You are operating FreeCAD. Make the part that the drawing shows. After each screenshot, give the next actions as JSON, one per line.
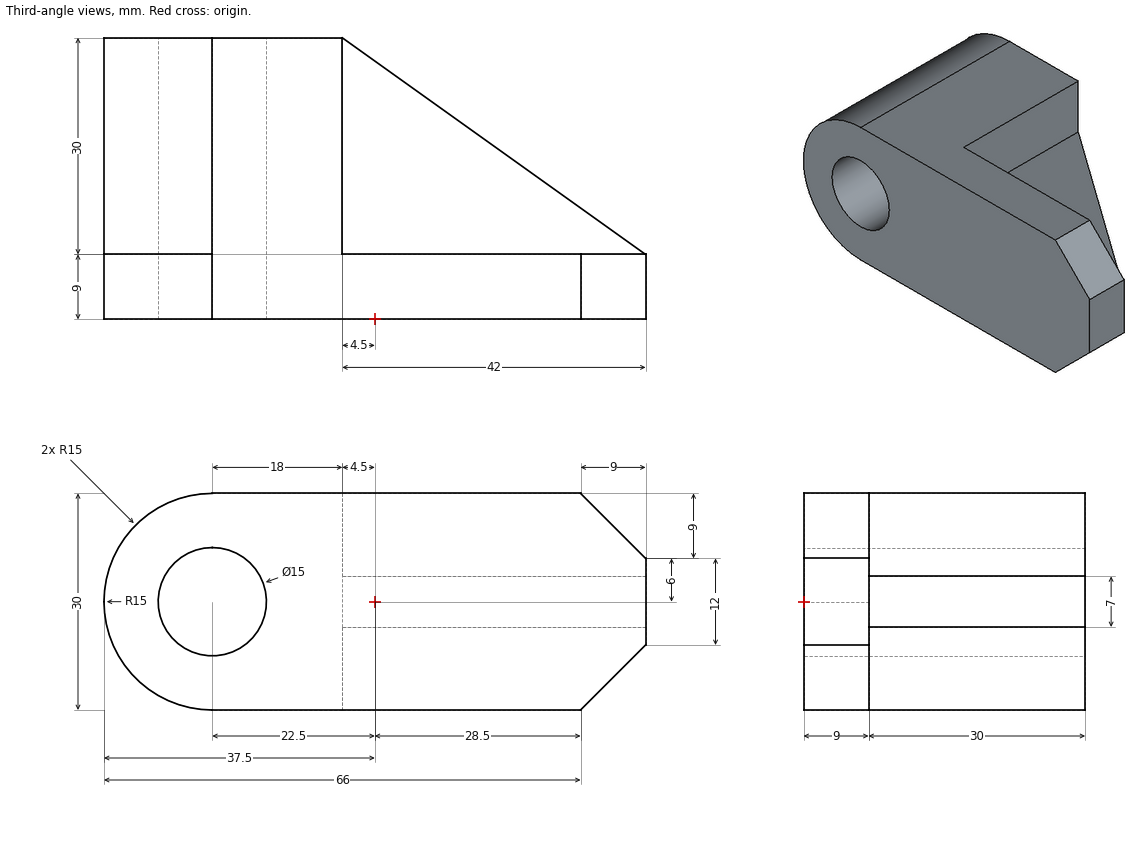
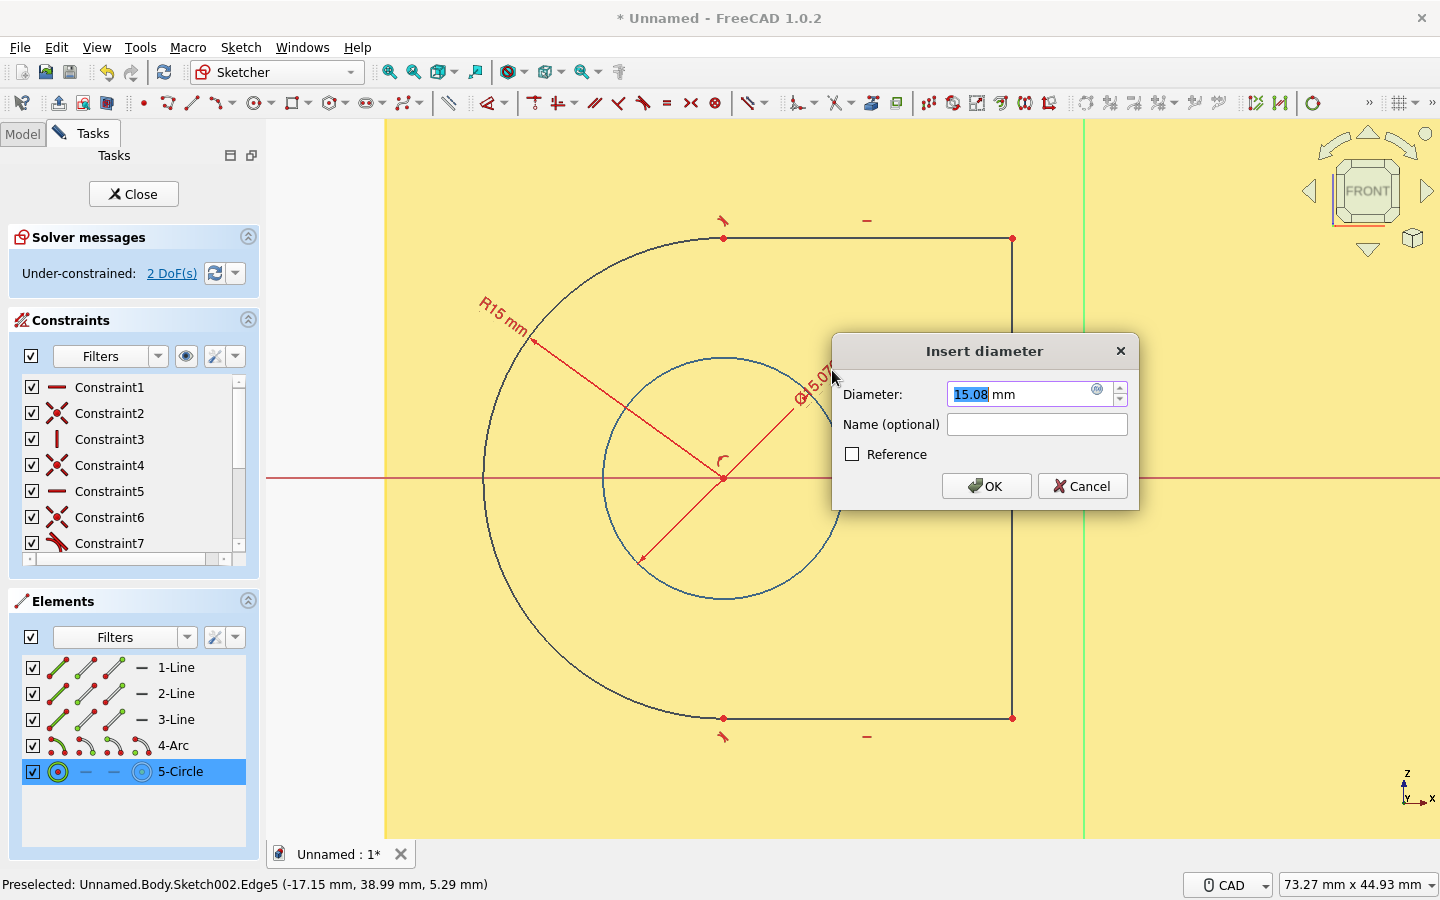
{"action": "type", "text": "15"}
{"action": "key", "text": "Return"}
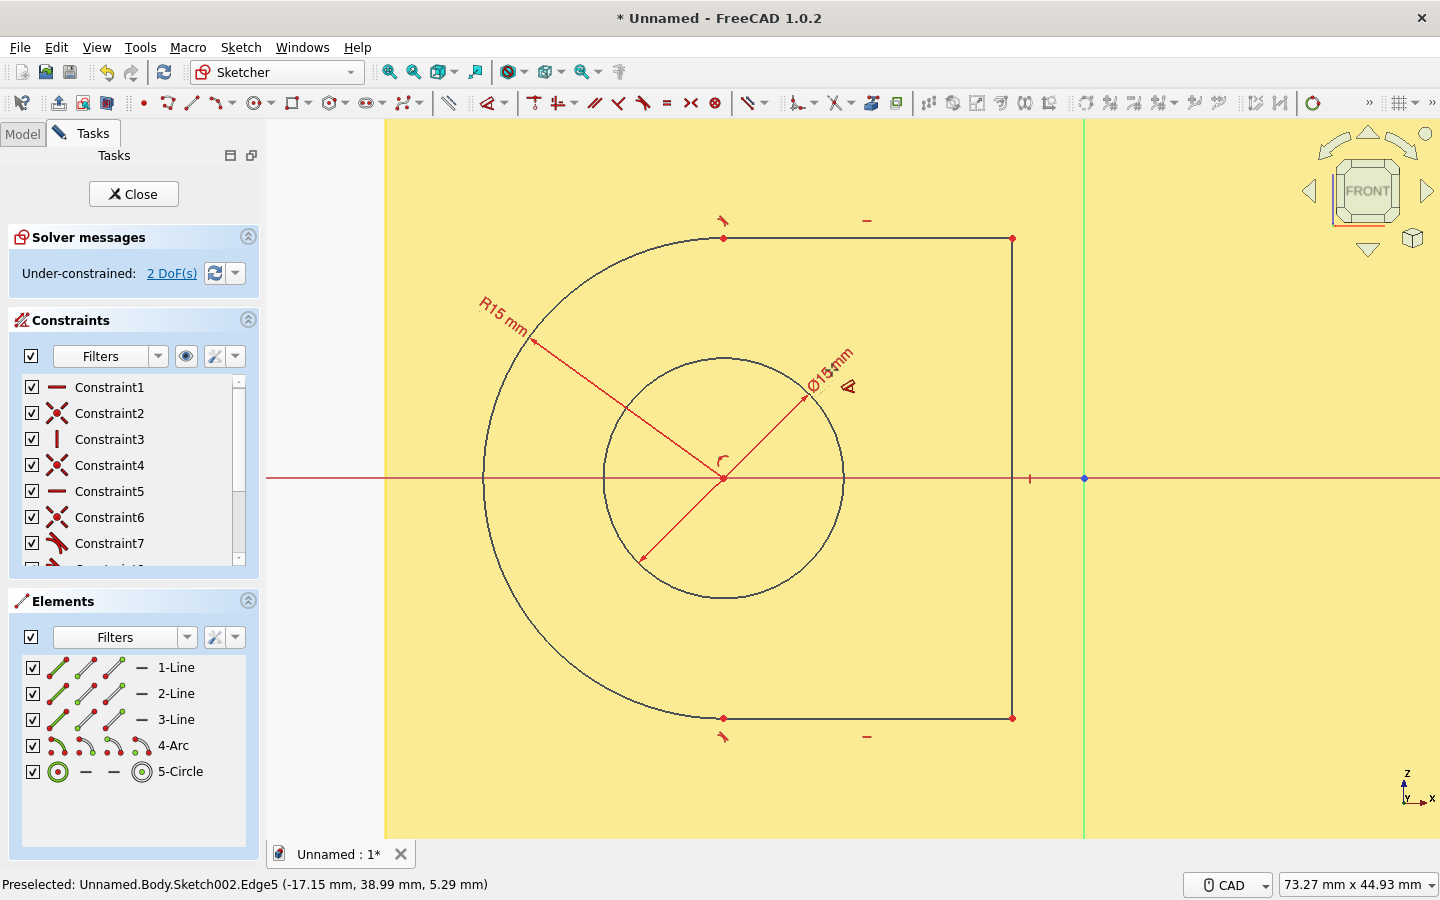
{"action": "left_click", "coordinate": [810, 238]}
{"action": "left_click", "coordinate": [868, 204]}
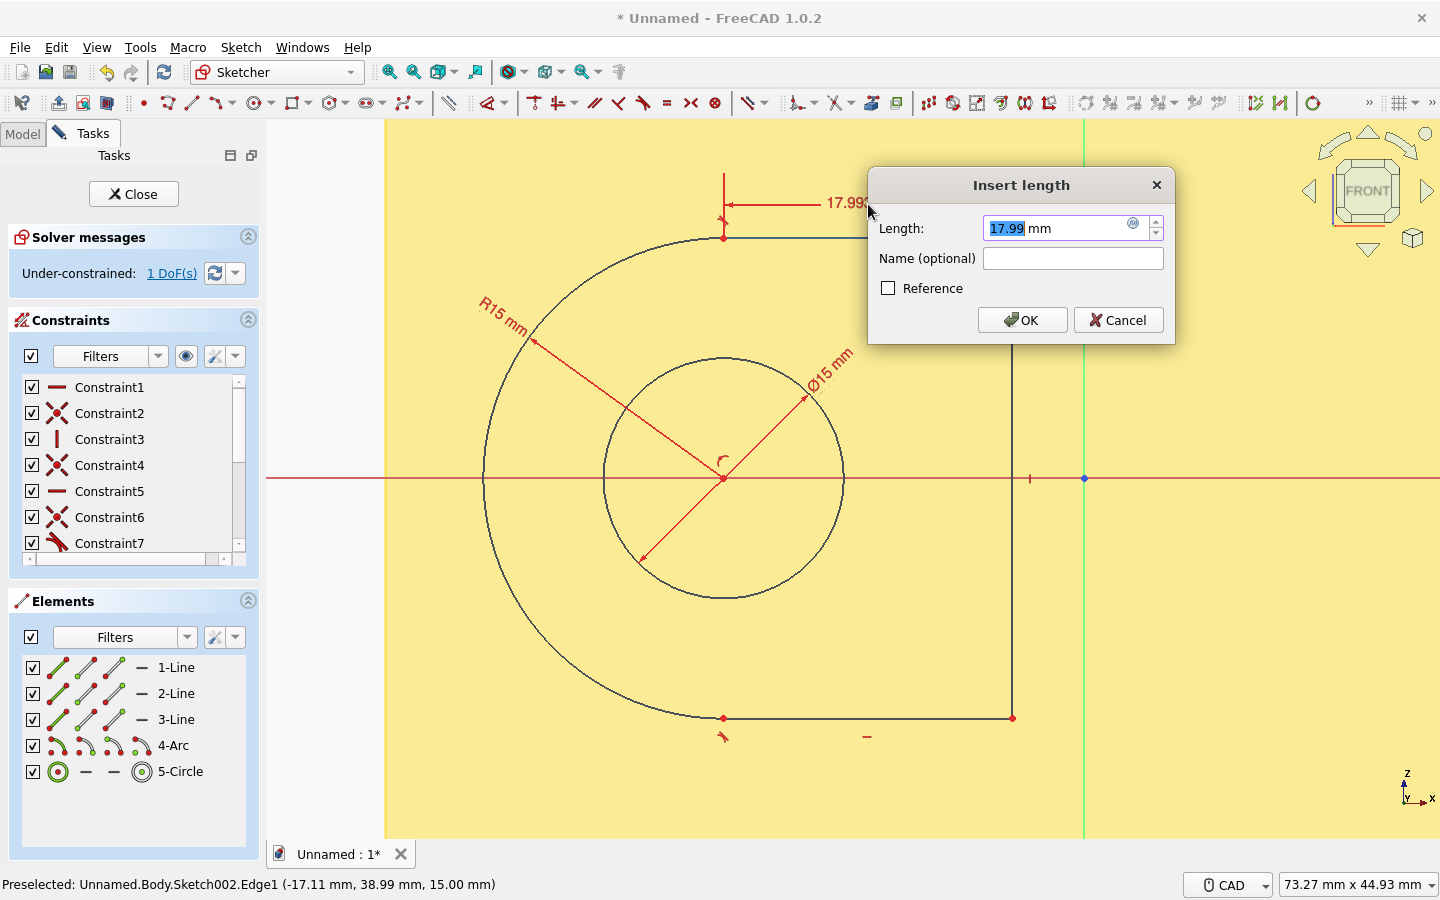
{"action": "type", "text": "18"}
{"action": "key", "text": "Return"}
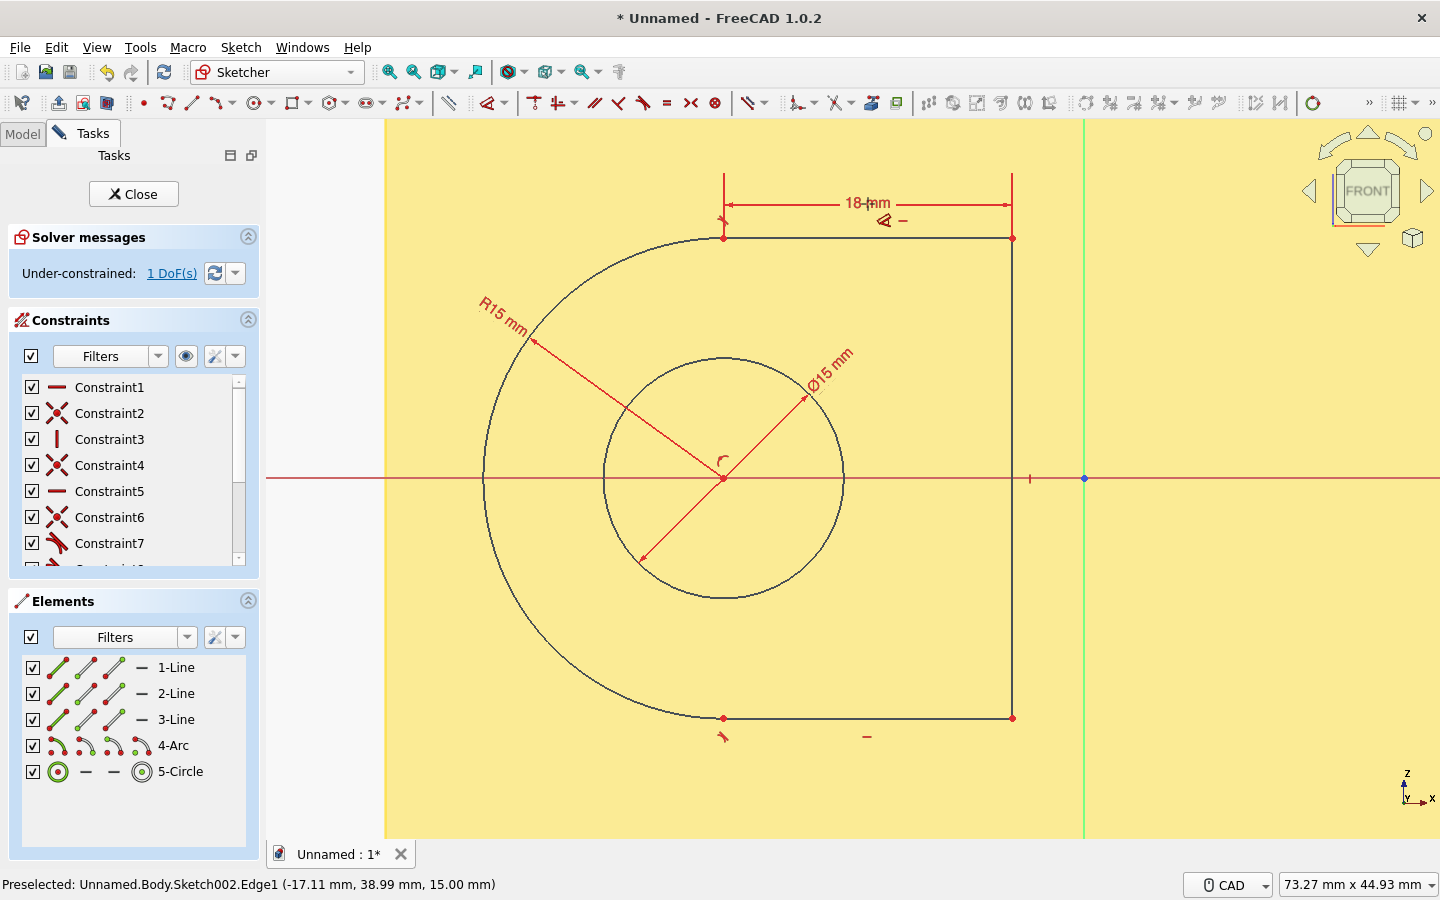
{"action": "left_click", "coordinate": [1012, 238]}
{"action": "left_click", "coordinate": [1048, 204]}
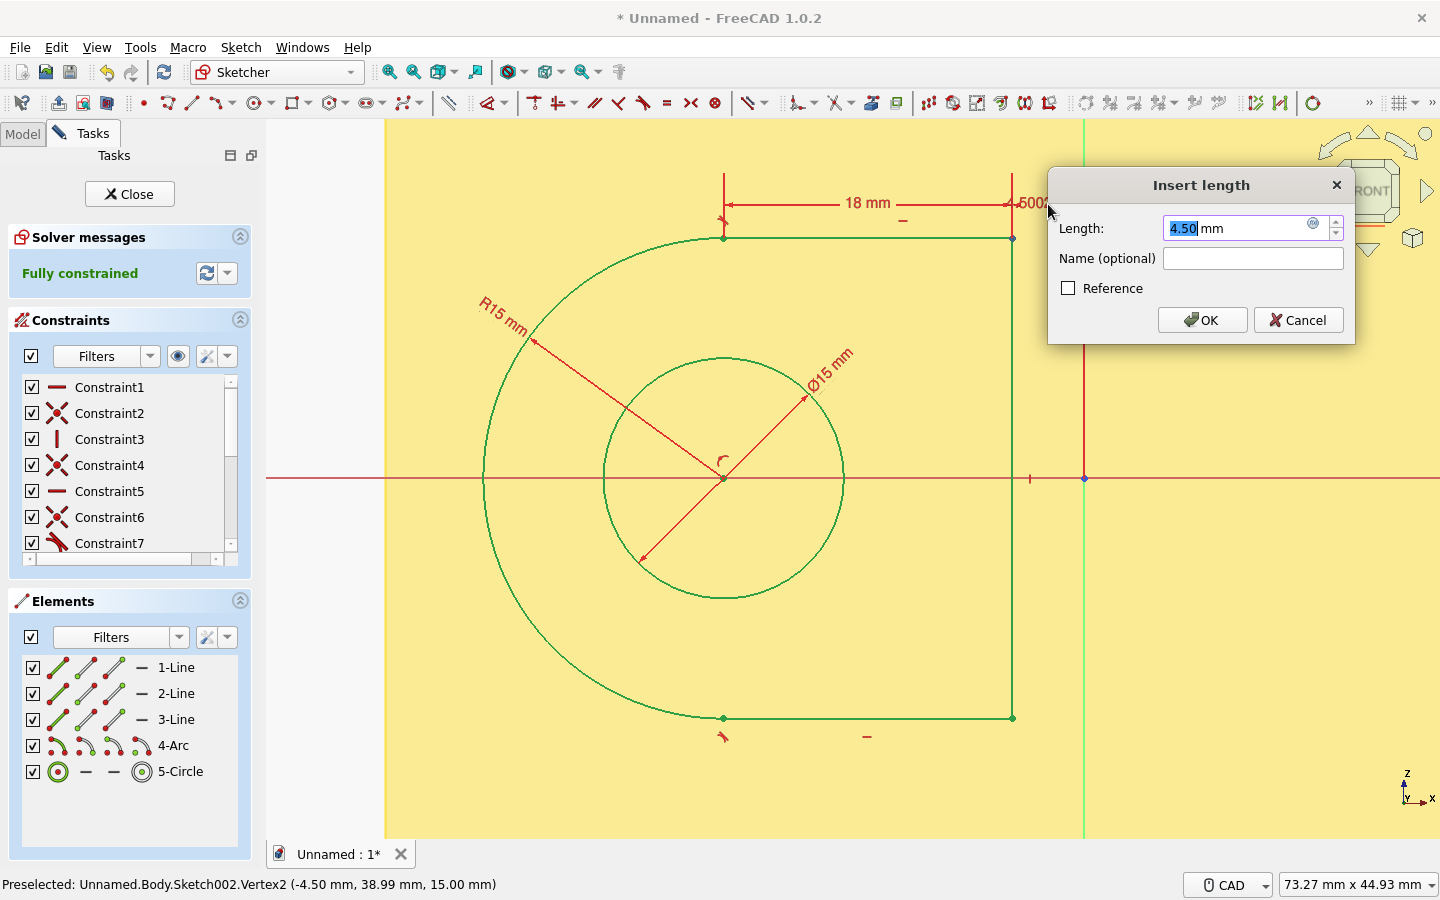
{"action": "type", "text": "4.5"}
{"action": "key", "text": "Return"}
{"action": "key", "text": "Escape"}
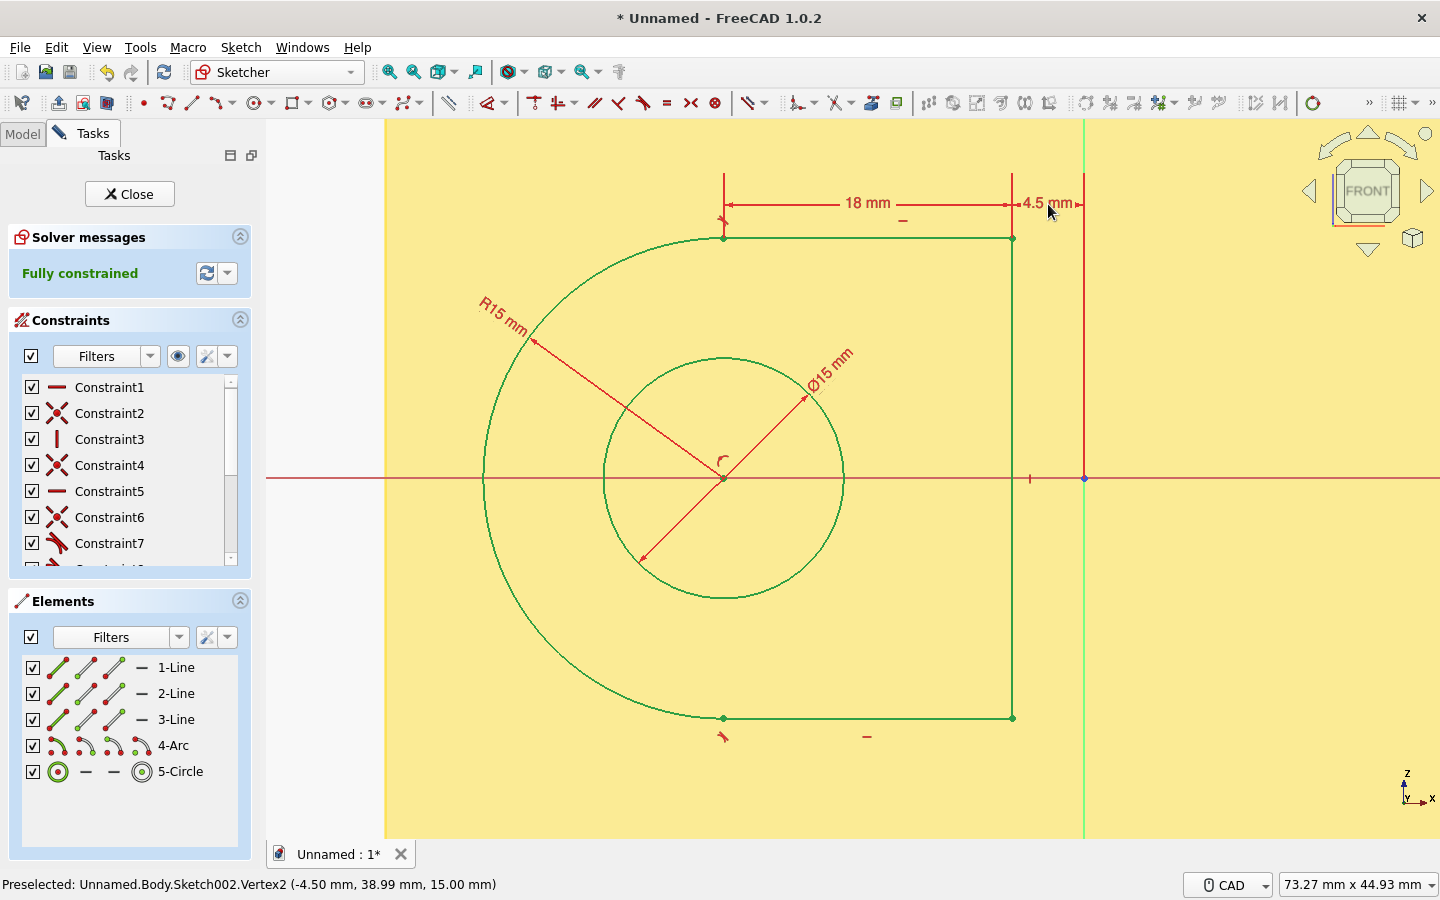
{"action": "left_click", "coordinate": [130, 194]}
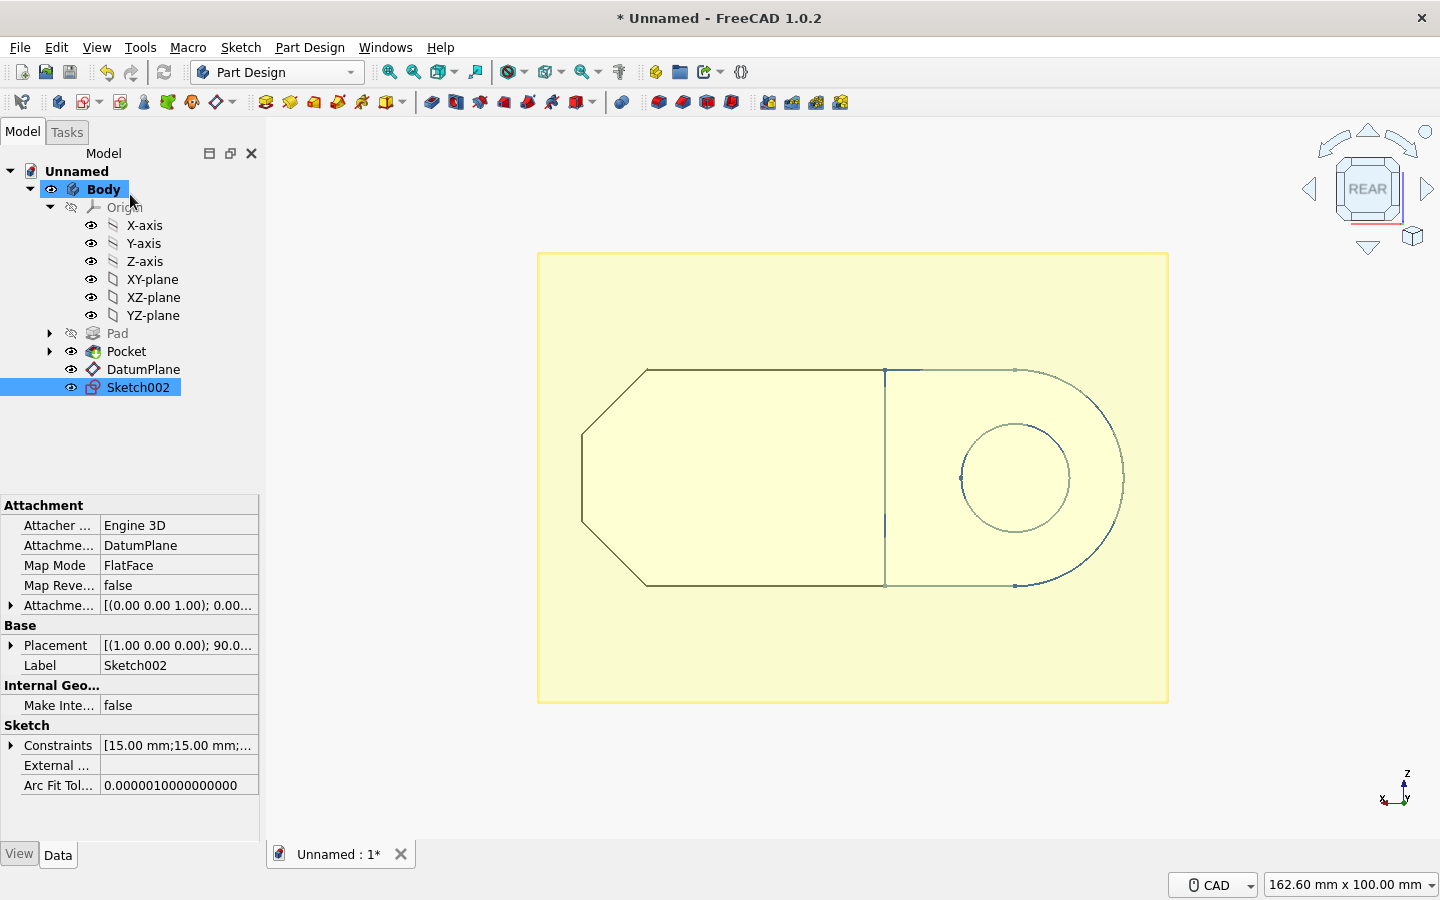
{"action": "left_click", "coordinate": [266, 102]}